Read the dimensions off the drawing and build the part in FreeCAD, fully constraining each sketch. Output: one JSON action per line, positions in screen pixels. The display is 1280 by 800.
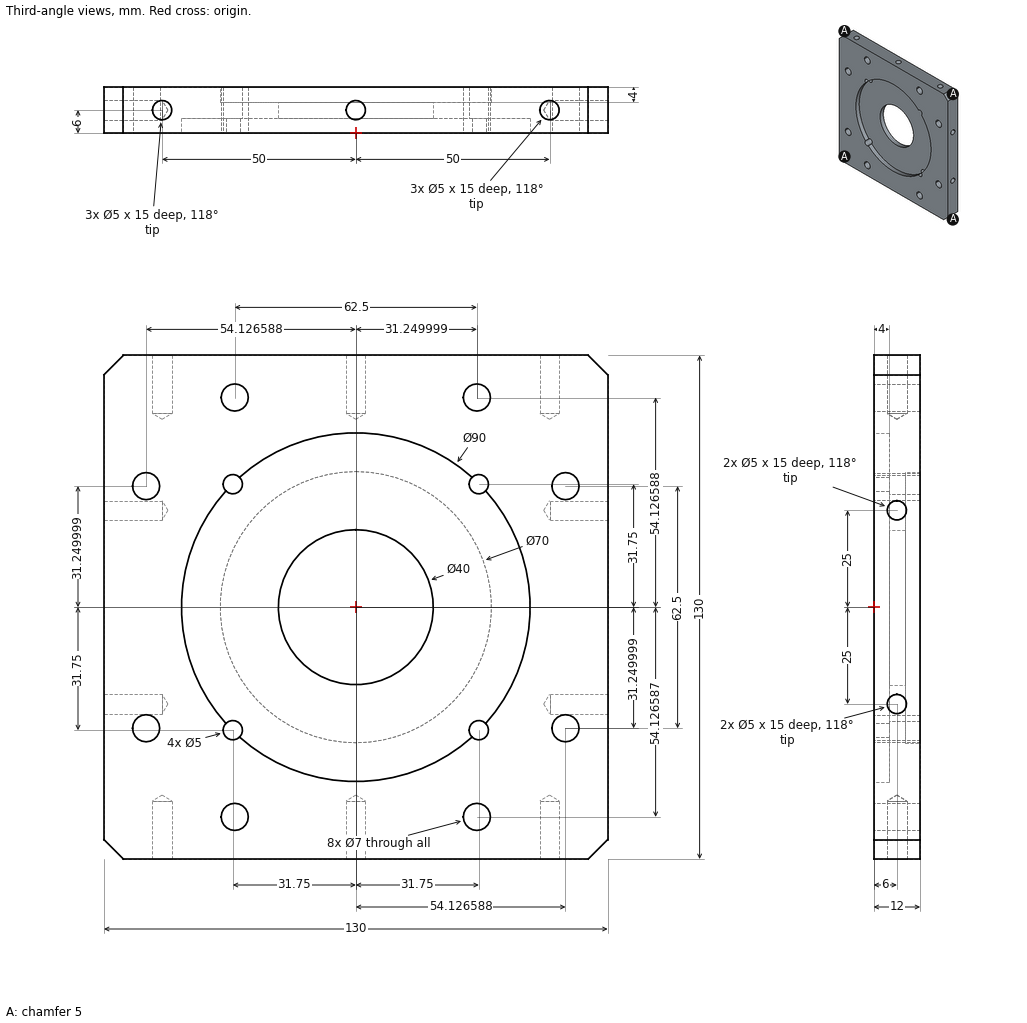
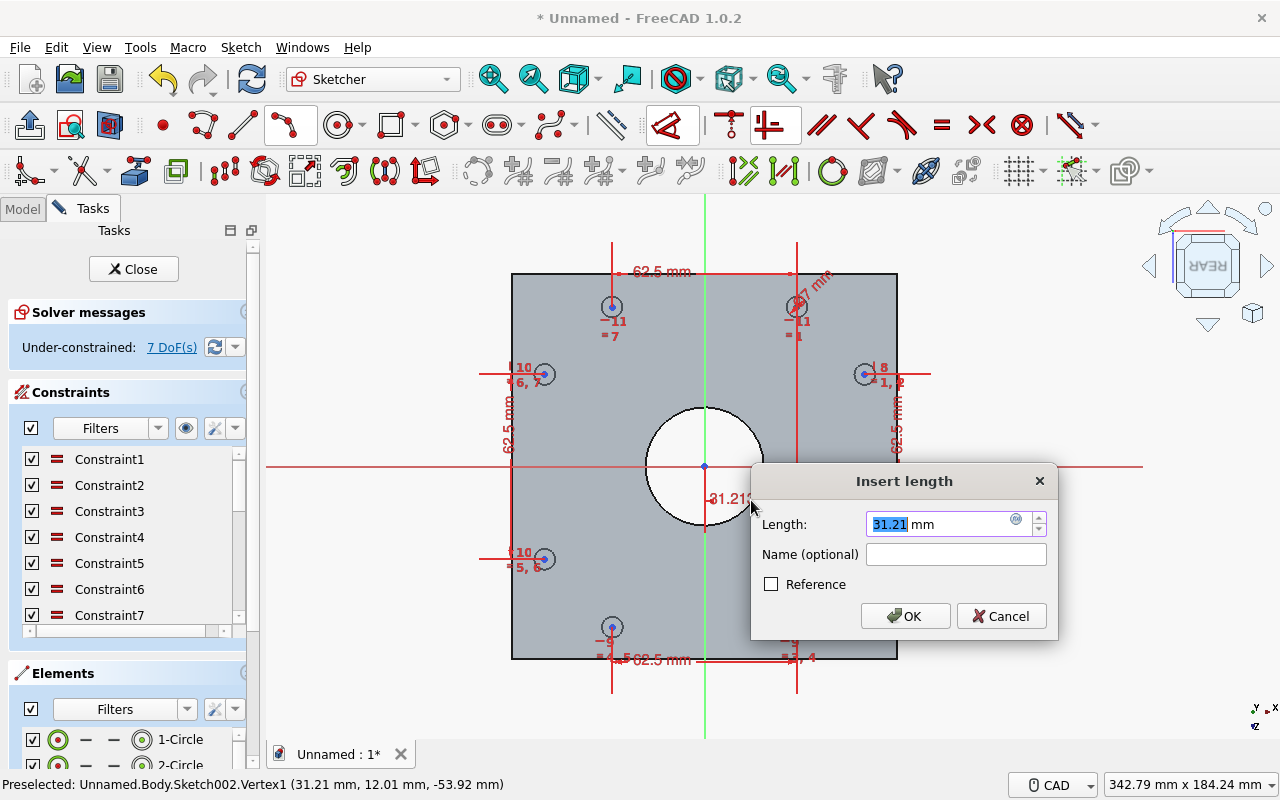
{"action": "type", "text": "31.250001"}
{"action": "key", "text": "Return"}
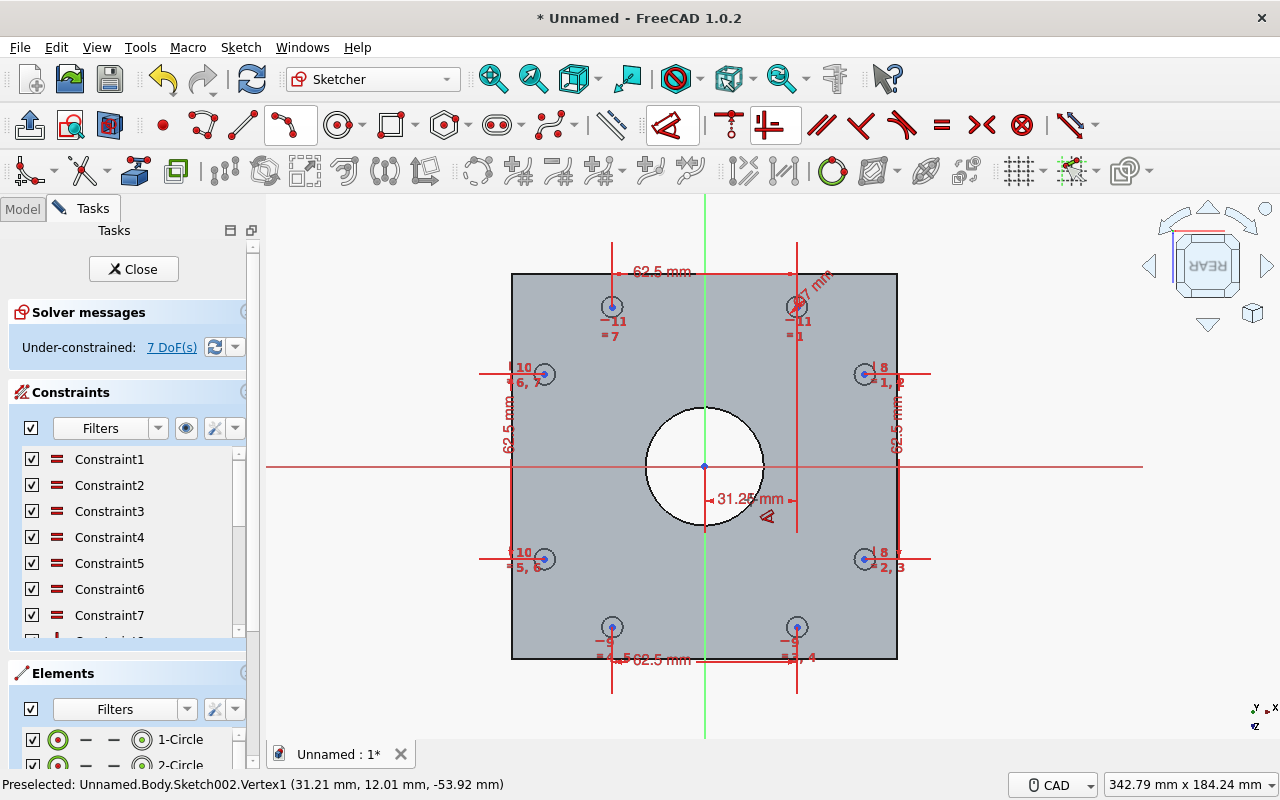
{"action": "left_click", "coordinate": [797, 307]}
{"action": "left_click", "coordinate": [831, 387]}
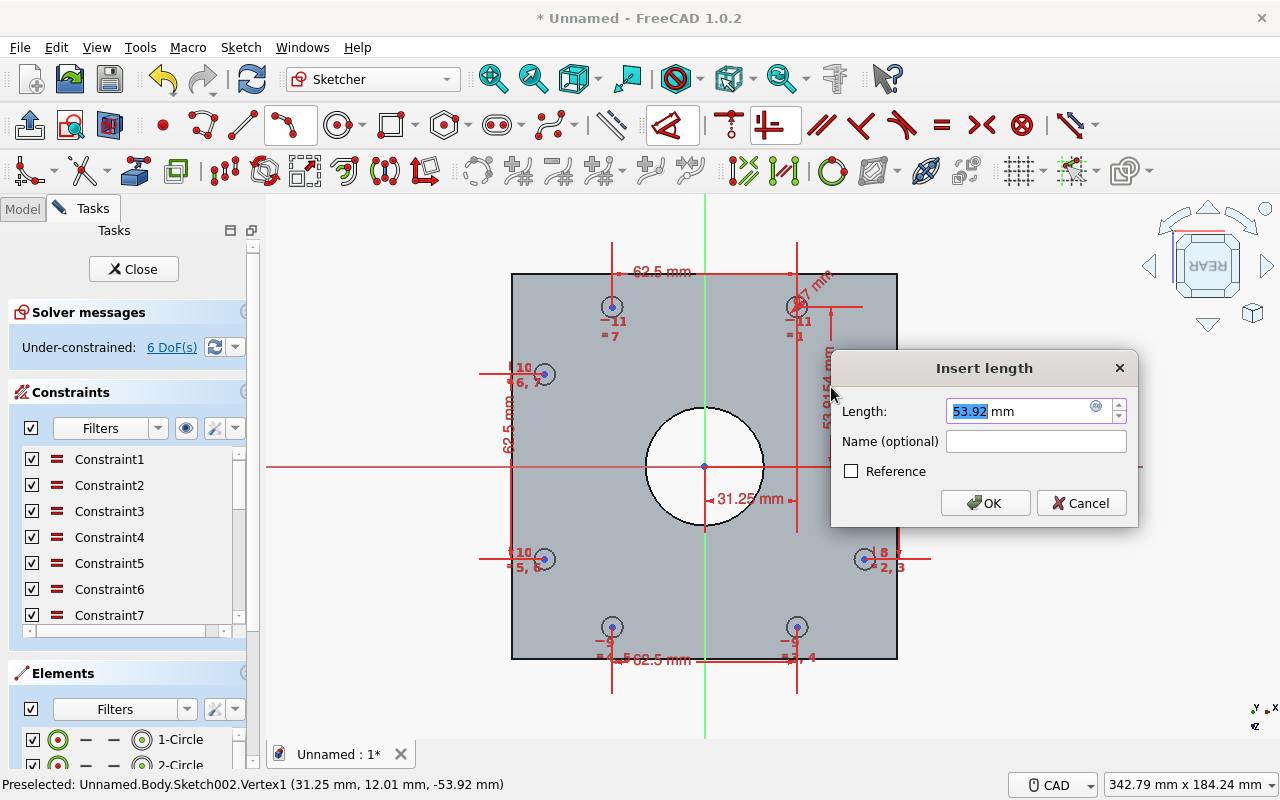
{"action": "type", "text": "54.126587"}
{"action": "key", "text": "Return"}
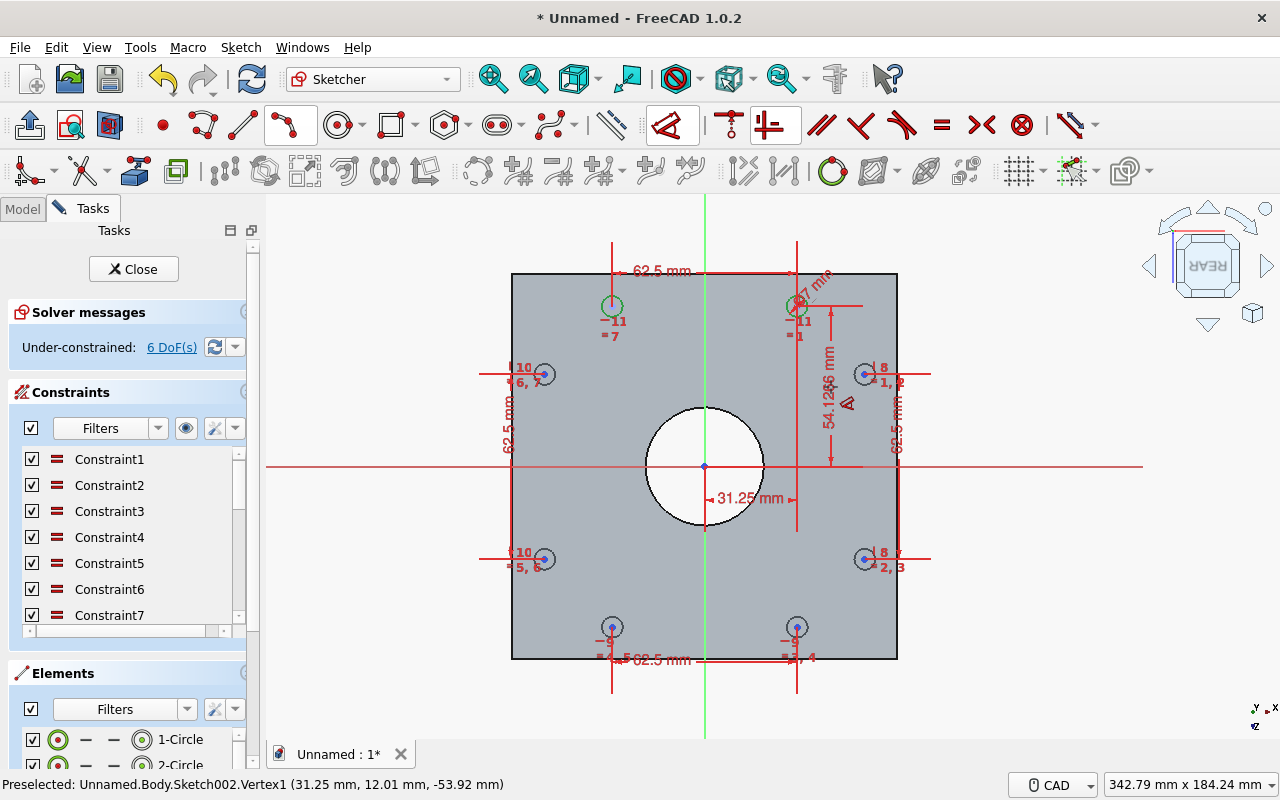
{"action": "left_click", "coordinate": [865, 374]}
{"action": "left_click", "coordinate": [785, 340]}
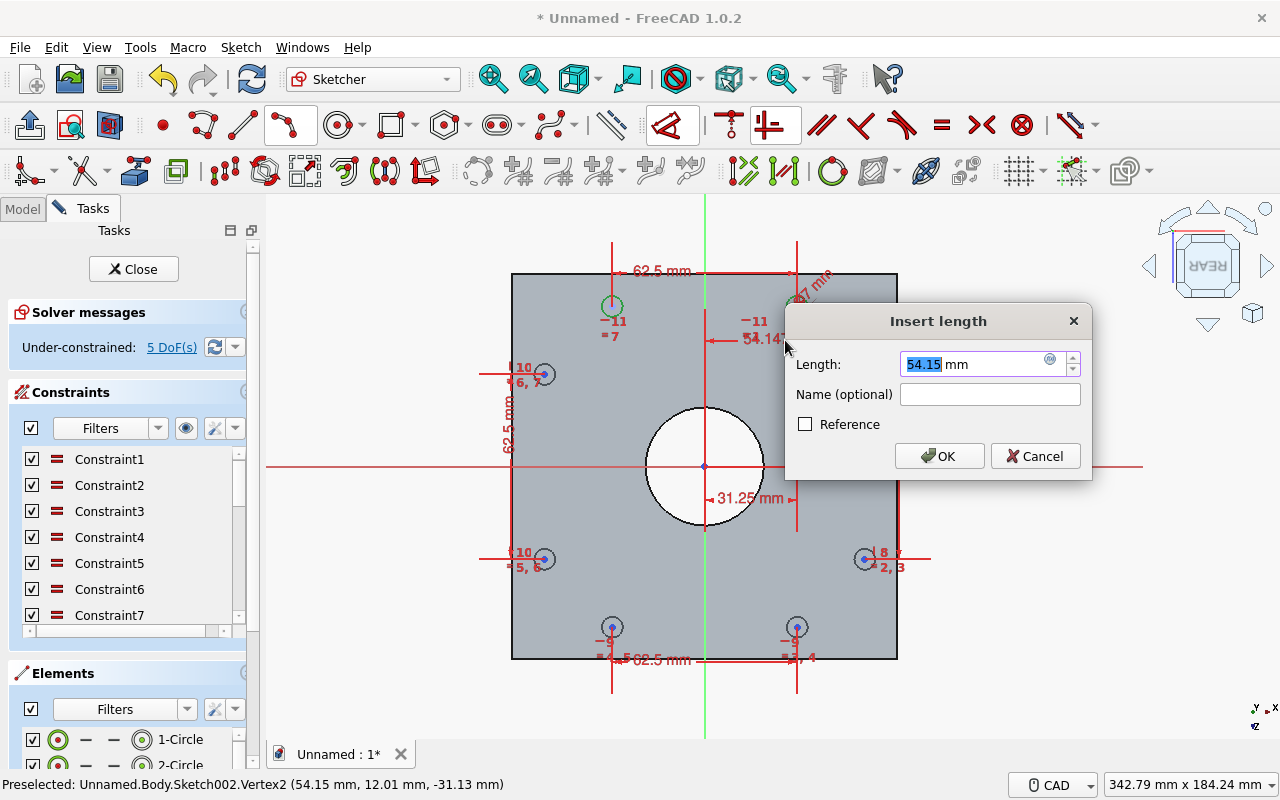
{"action": "type", "text": "54.126588"}
{"action": "key", "text": "Return"}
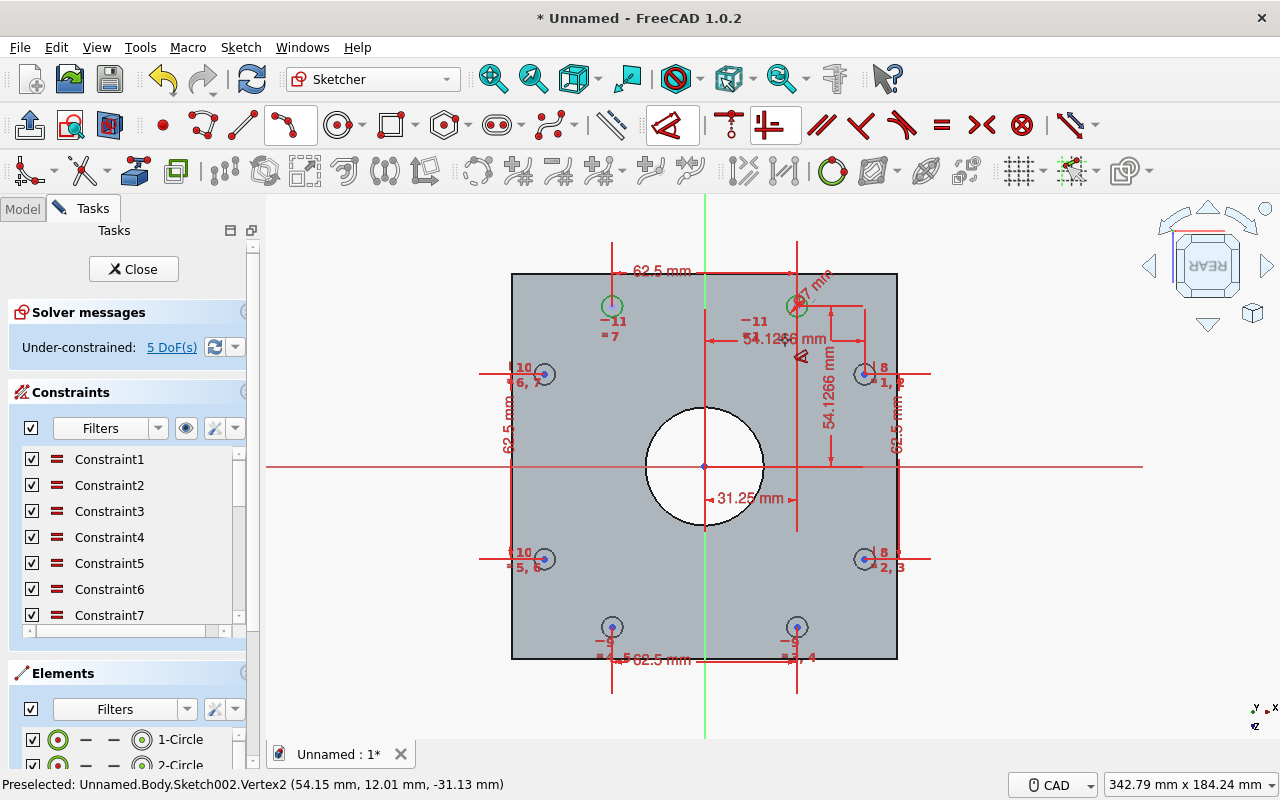
{"action": "left_click", "coordinate": [865, 374]}
{"action": "left_click", "coordinate": [899, 453]}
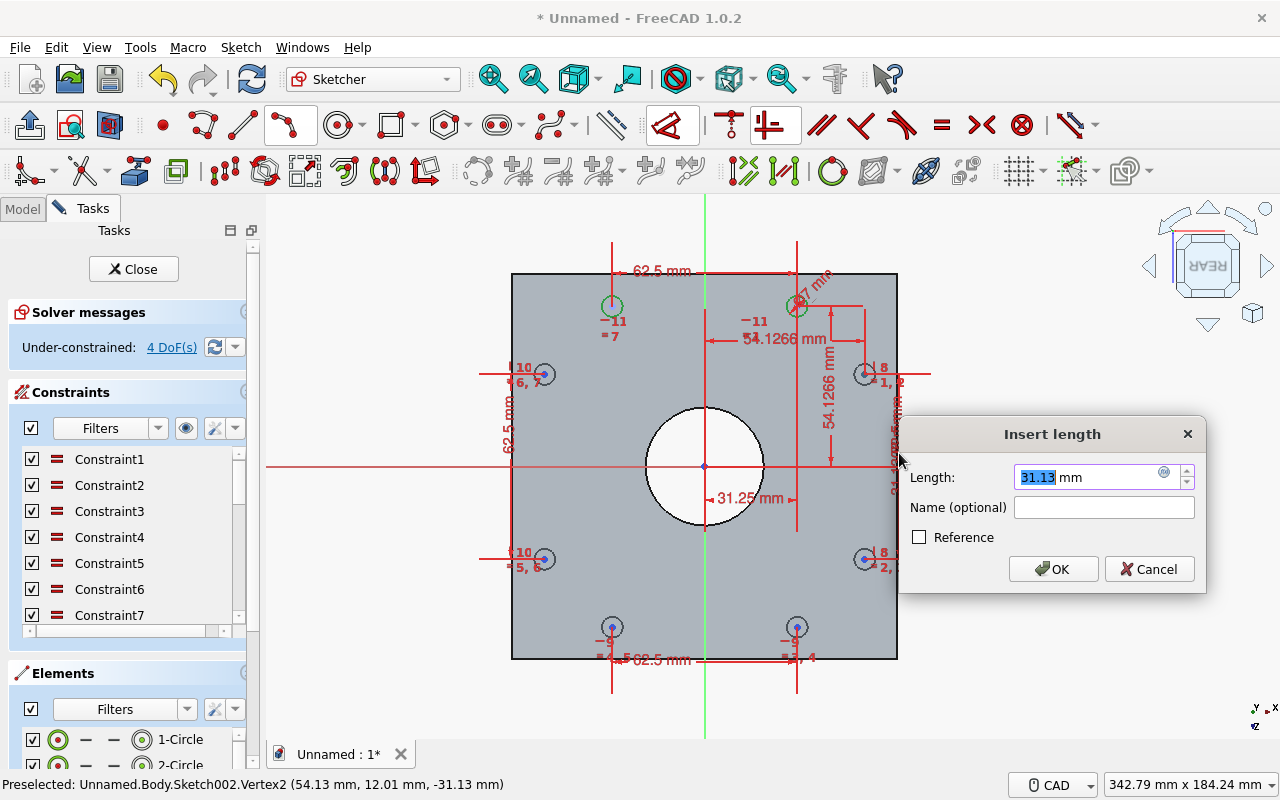
{"action": "type", "text": "31.249999"}
{"action": "key", "text": "Return"}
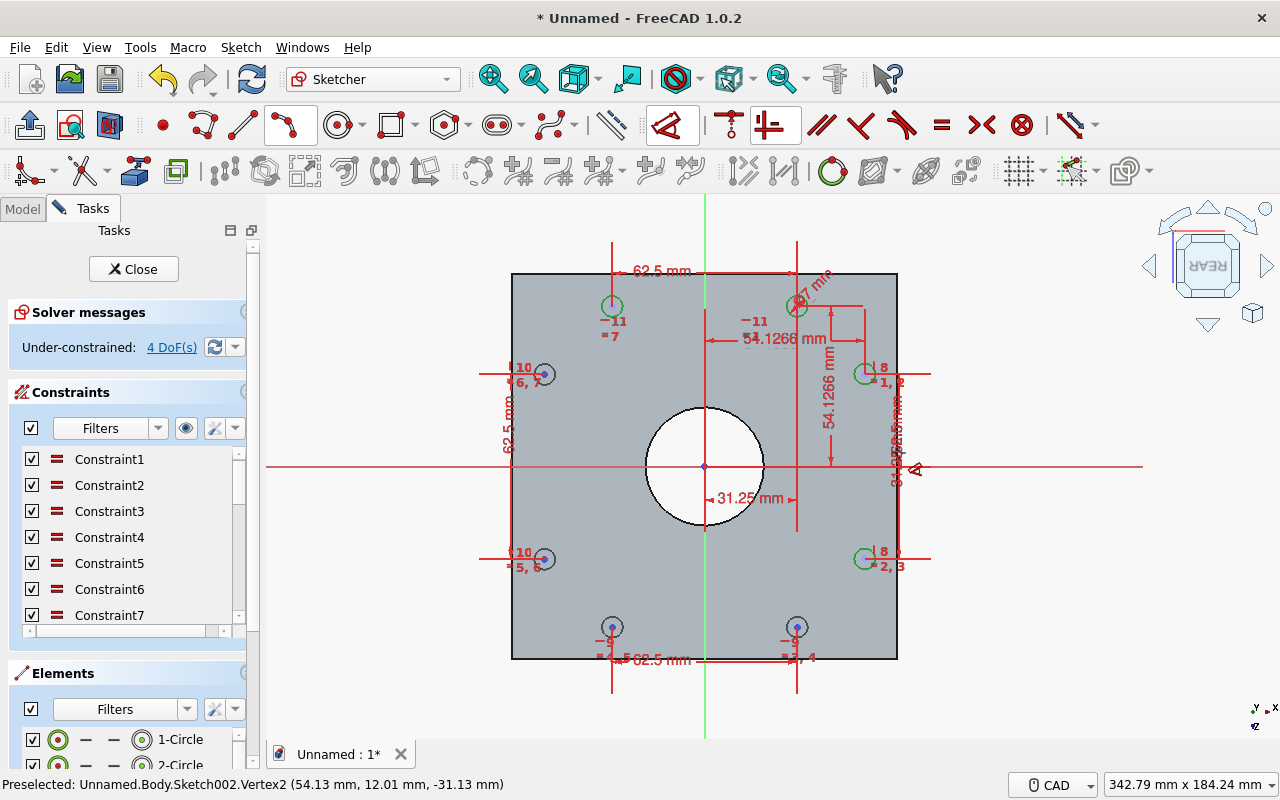
{"action": "left_click", "coordinate": [797, 627]}
{"action": "left_click", "coordinate": [751, 661]}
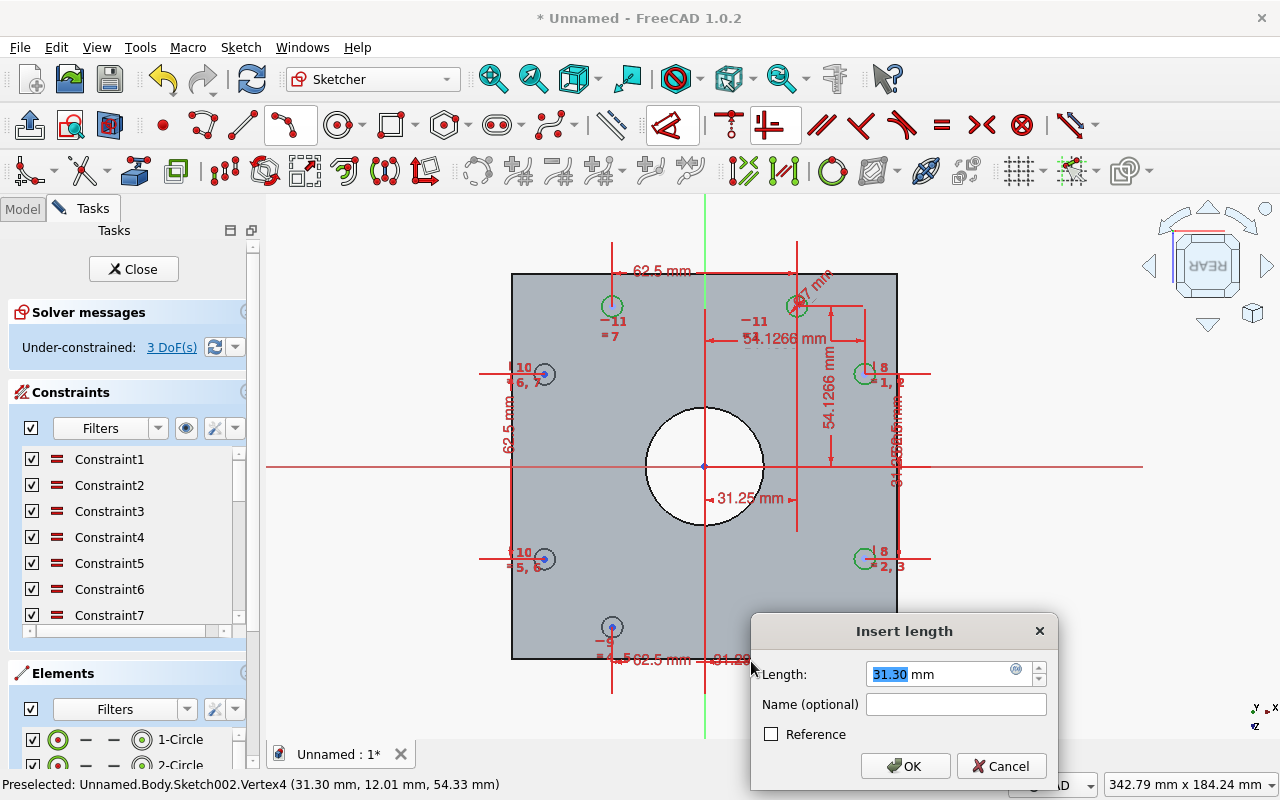
{"action": "type", "text": "31.249999"}
{"action": "key", "text": "Return"}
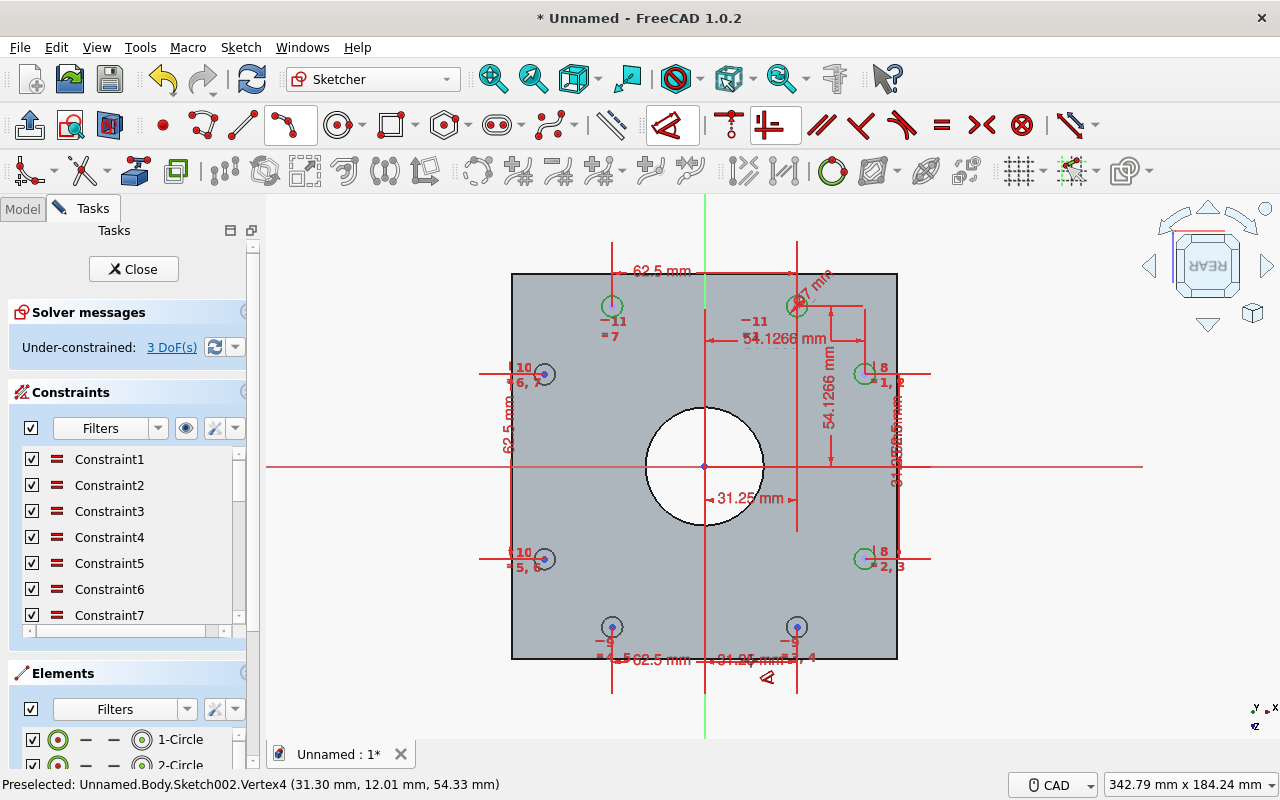
{"action": "left_click", "coordinate": [797, 627]}
{"action": "left_click", "coordinate": [831, 547]}